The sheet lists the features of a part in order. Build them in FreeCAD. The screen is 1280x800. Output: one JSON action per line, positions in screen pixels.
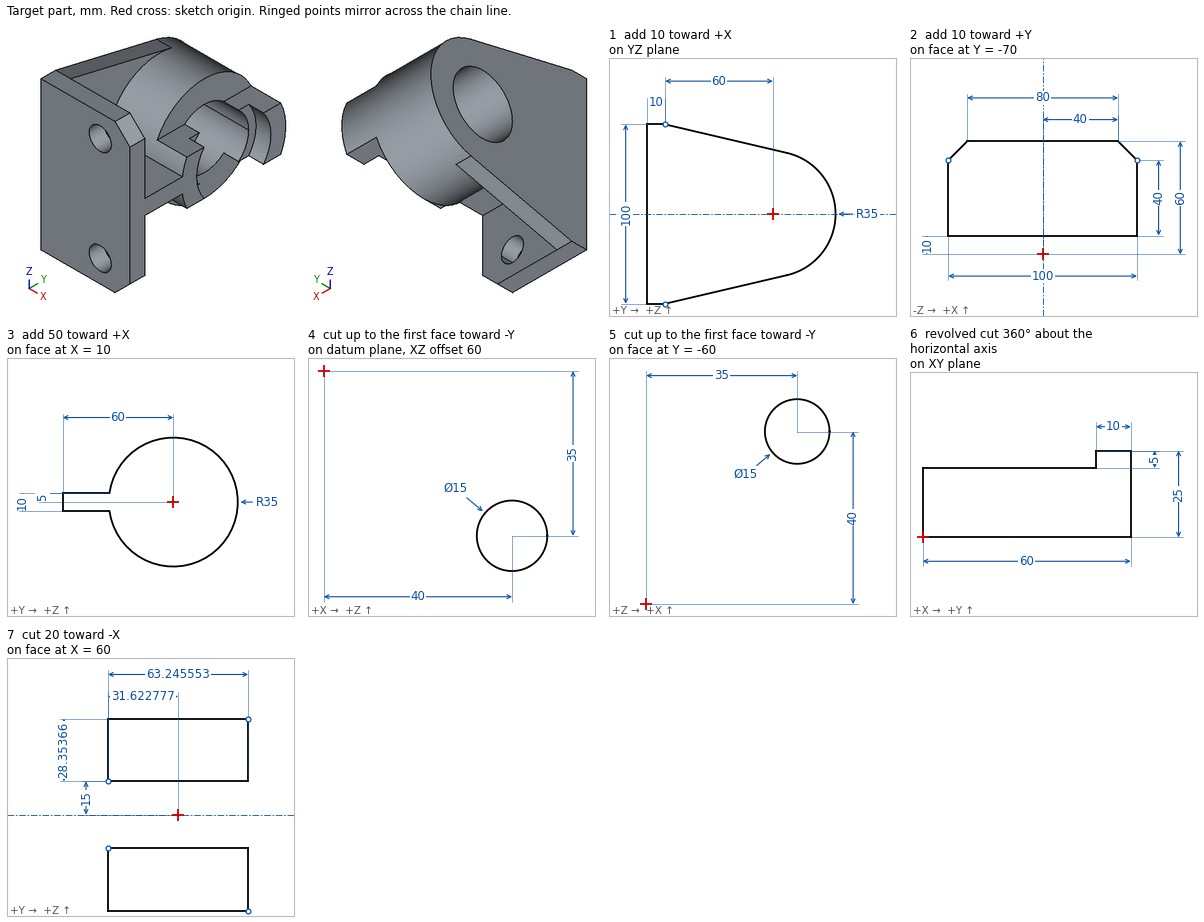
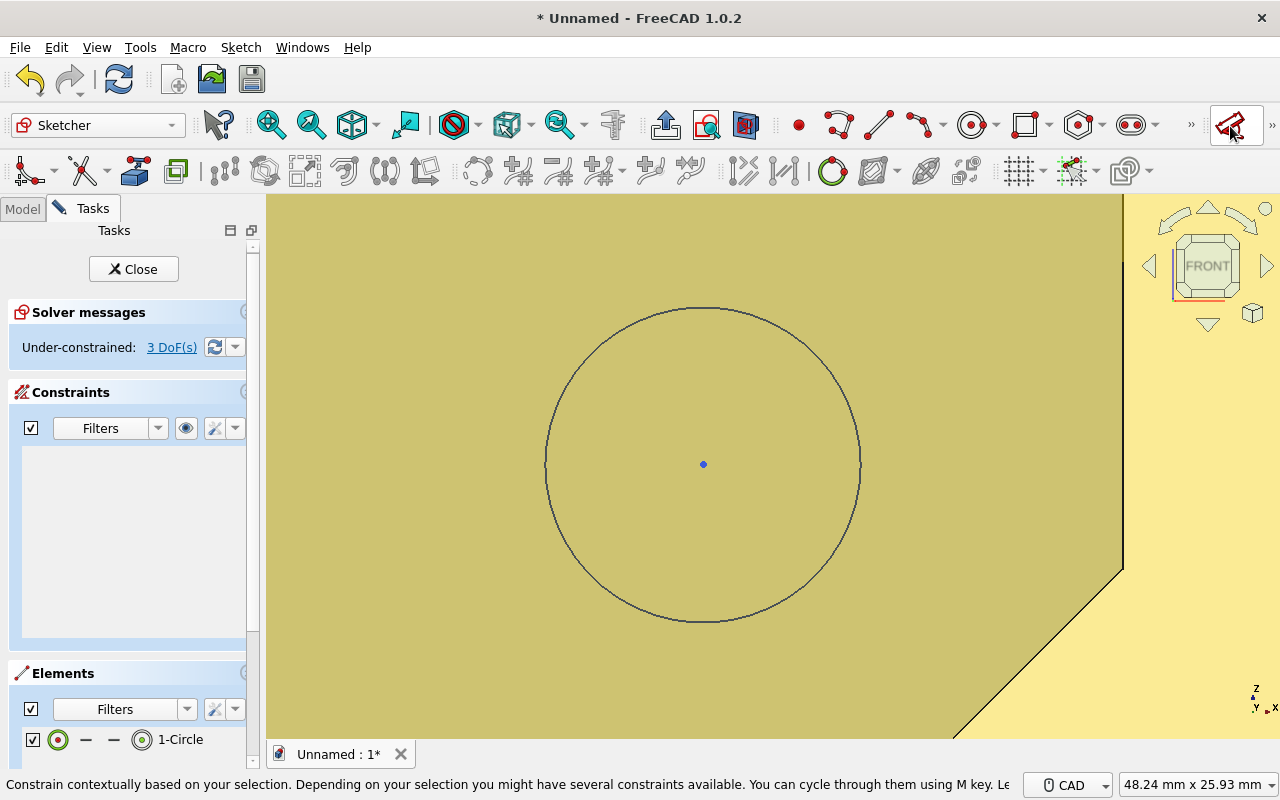
{"action": "left_click", "coordinate": [814, 353]}
{"action": "left_click", "coordinate": [837, 330]}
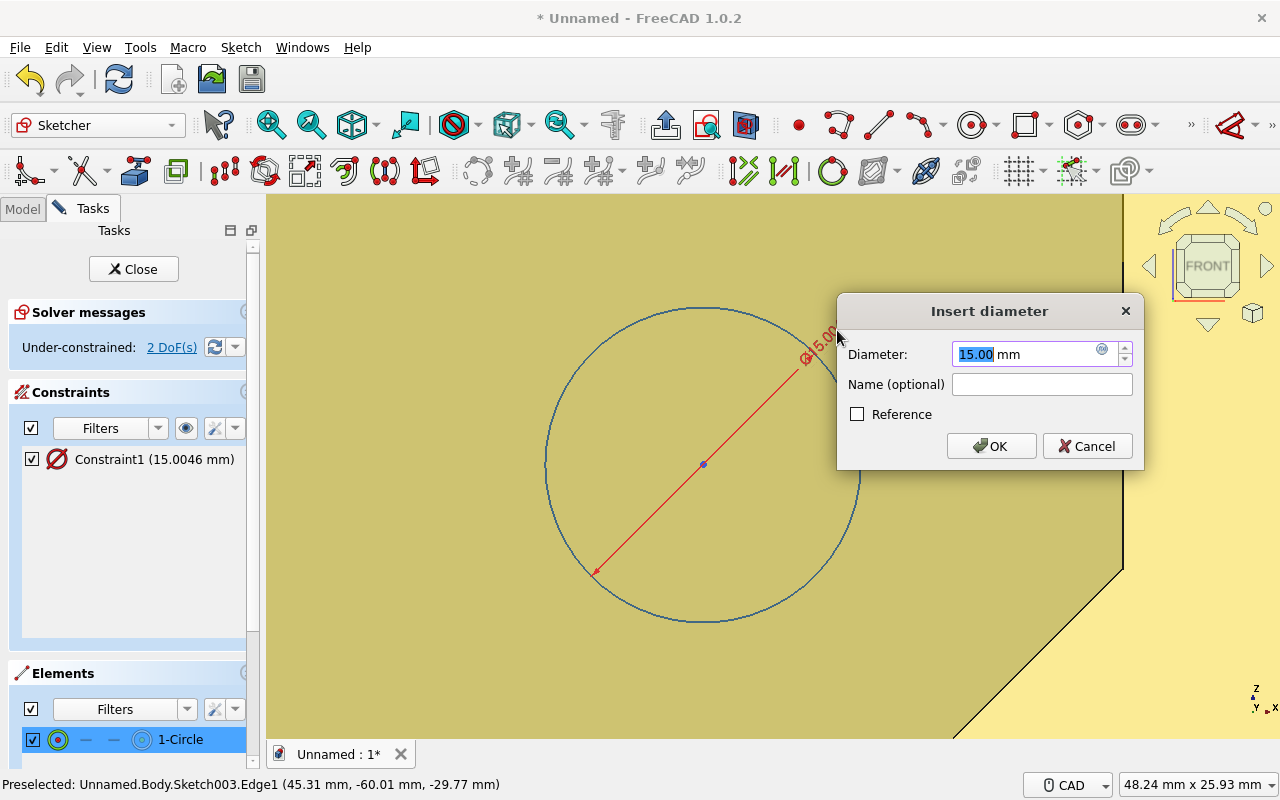
{"action": "type", "text": "15"}
{"action": "key", "text": "Return"}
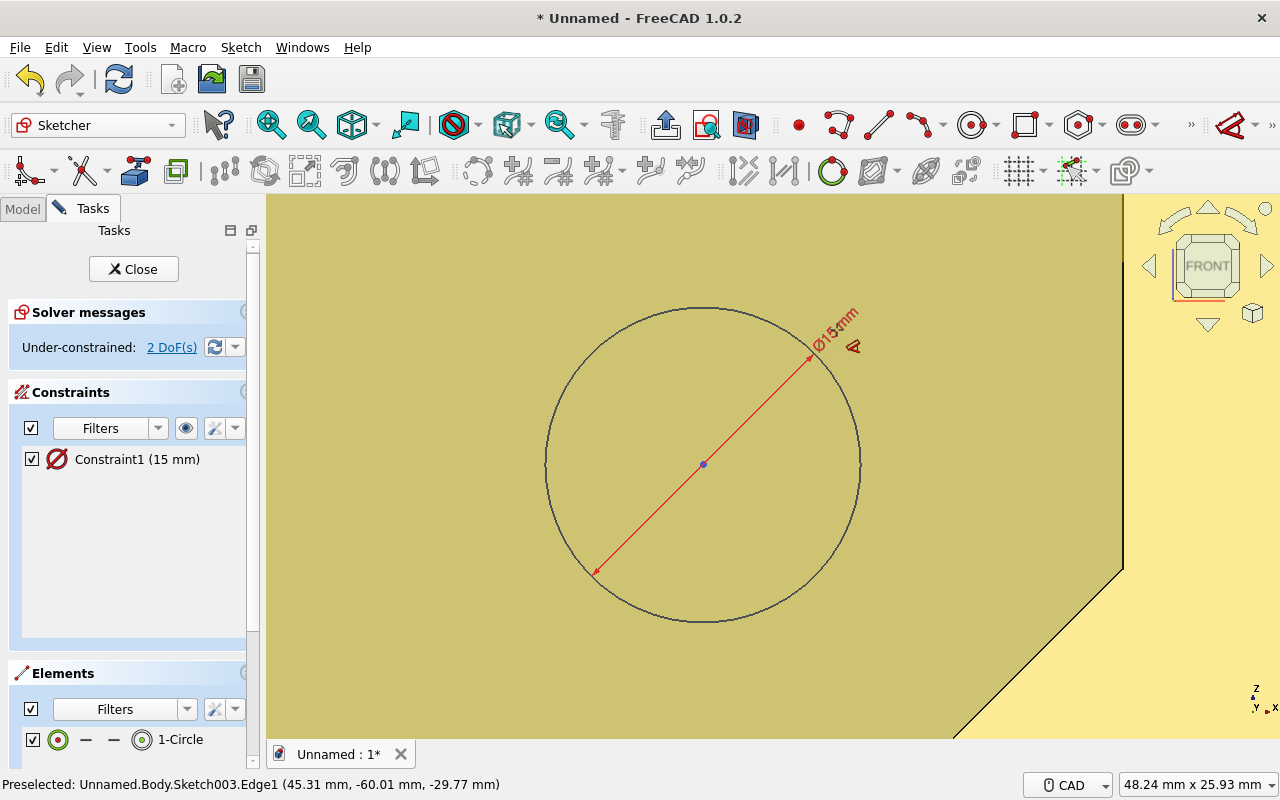
{"action": "left_click", "coordinate": [703, 465]}
{"action": "left_click", "coordinate": [498, 499]}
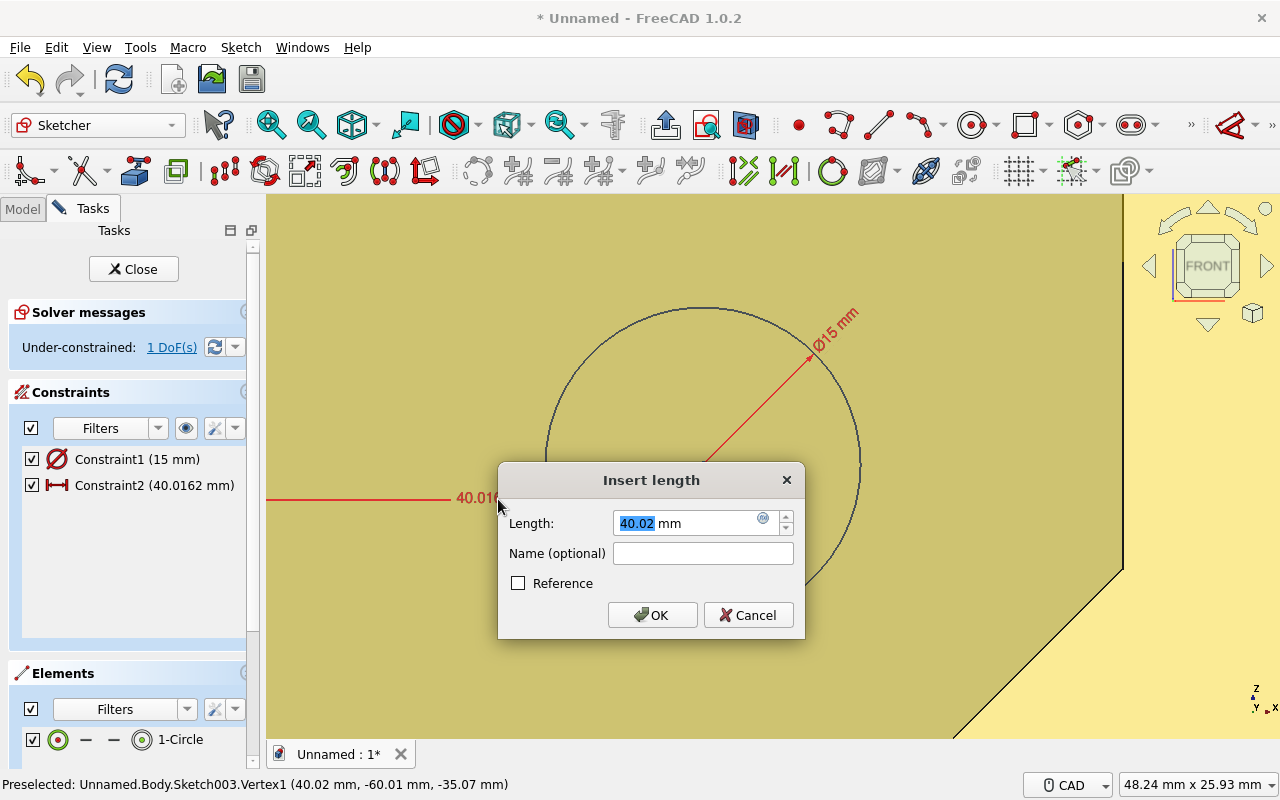
{"action": "type", "text": "40"}
{"action": "key", "text": "Return"}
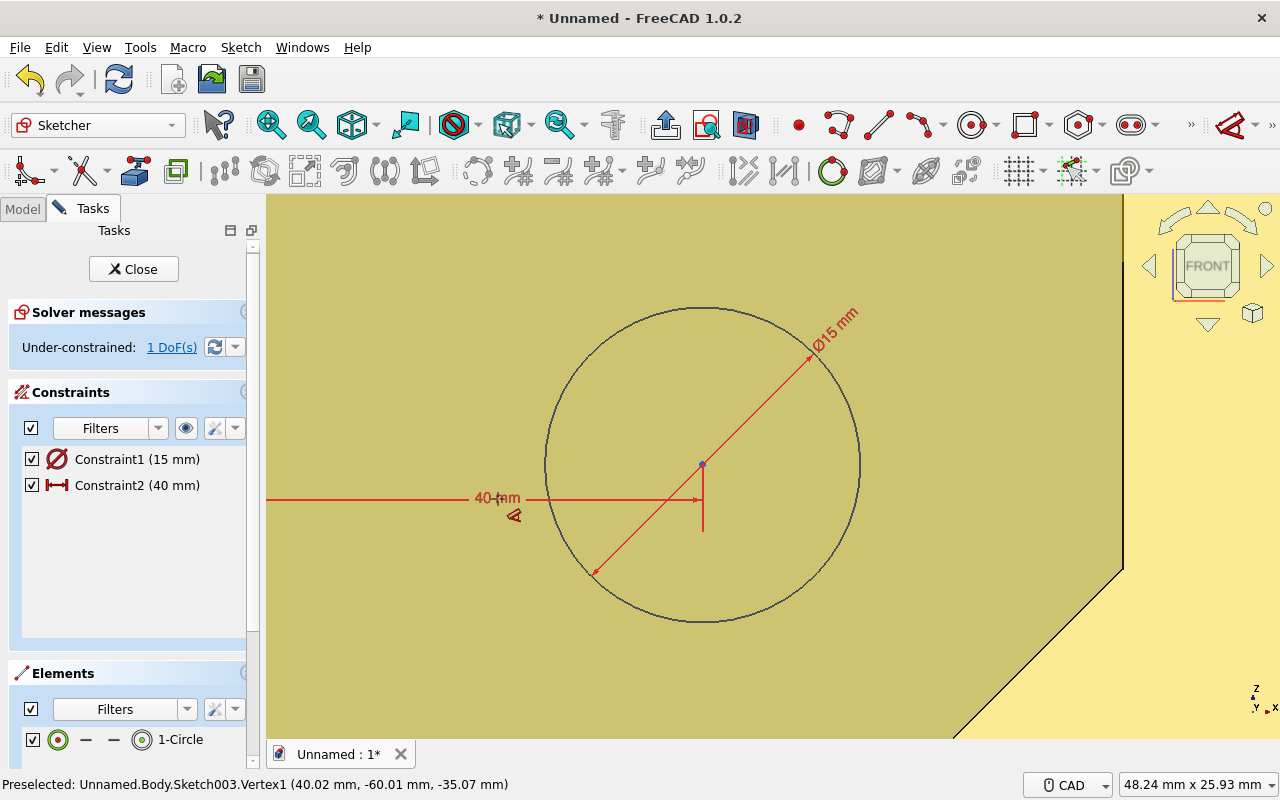
{"action": "left_click", "coordinate": [703, 465]}
{"action": "left_click", "coordinate": [737, 344]}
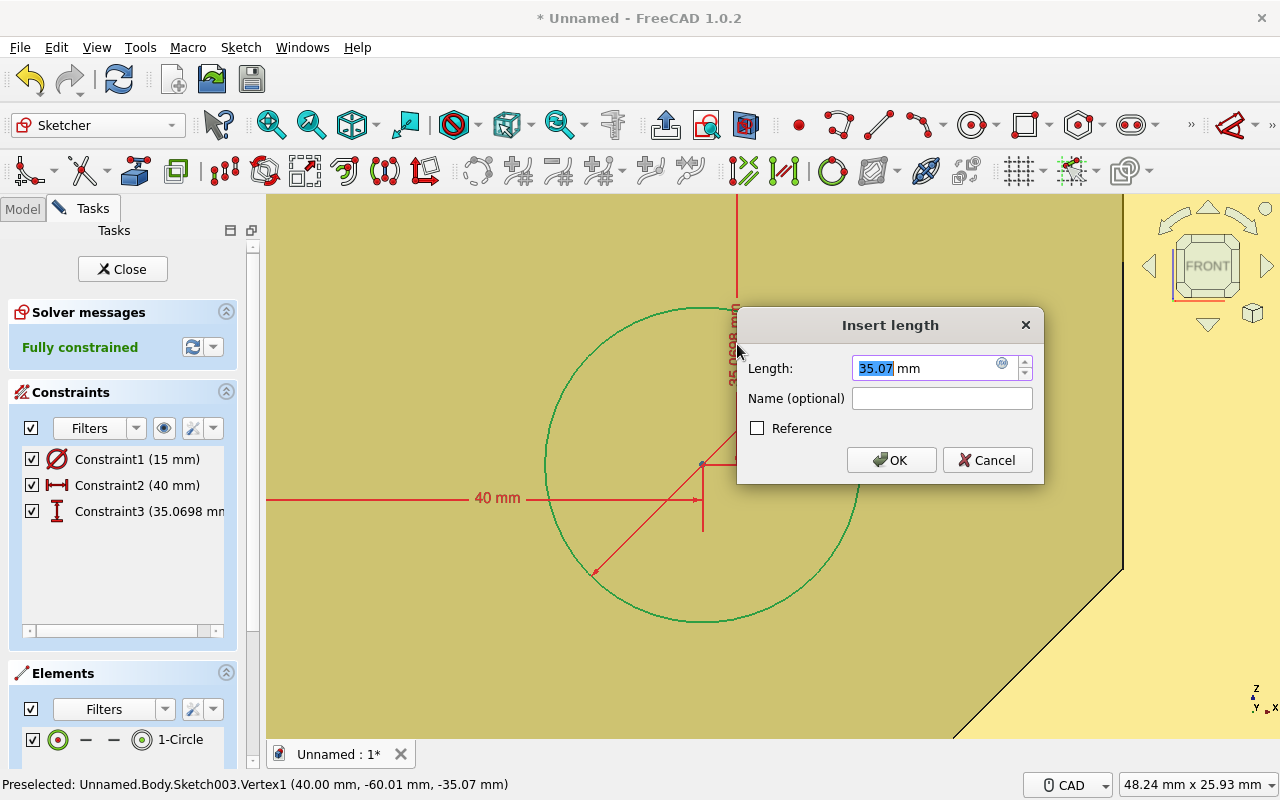
{"action": "type", "text": "35"}
{"action": "key", "text": "Return"}
{"action": "key", "text": "Escape"}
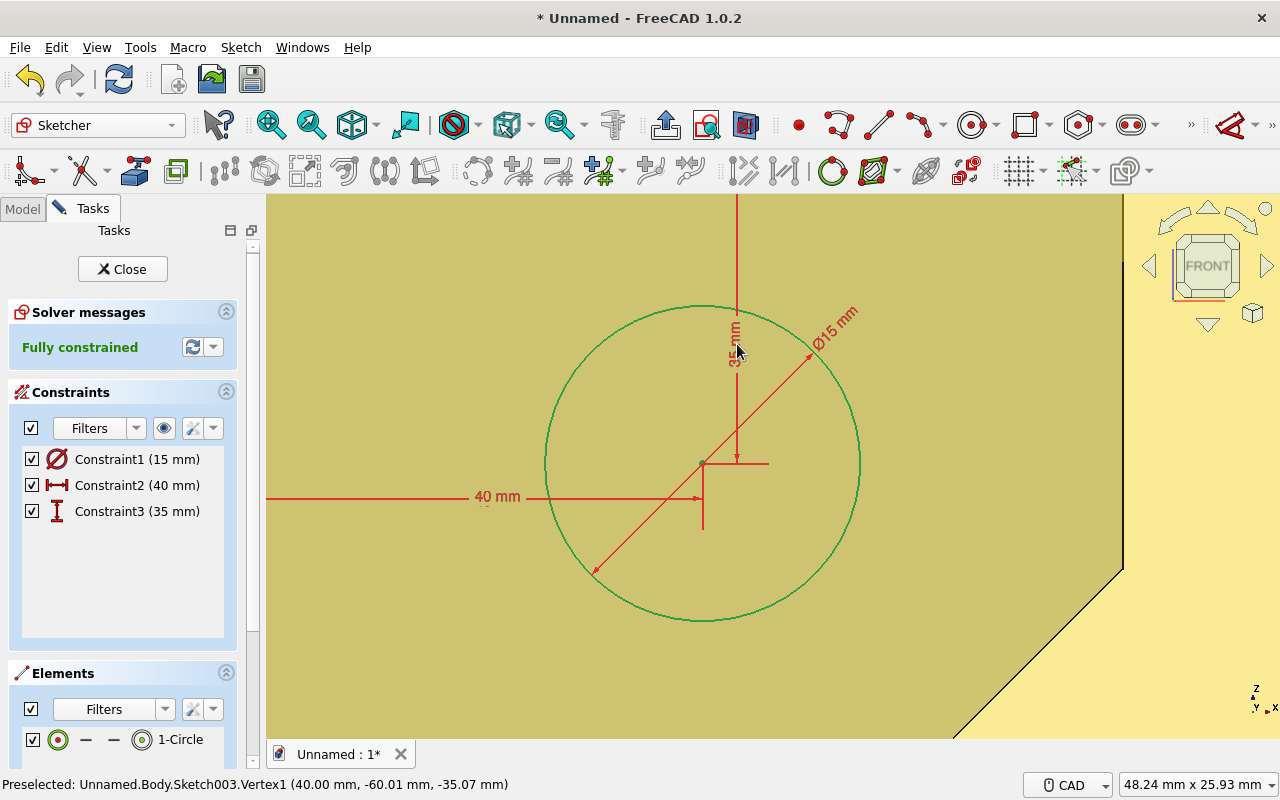
{"action": "left_click", "coordinate": [123, 269]}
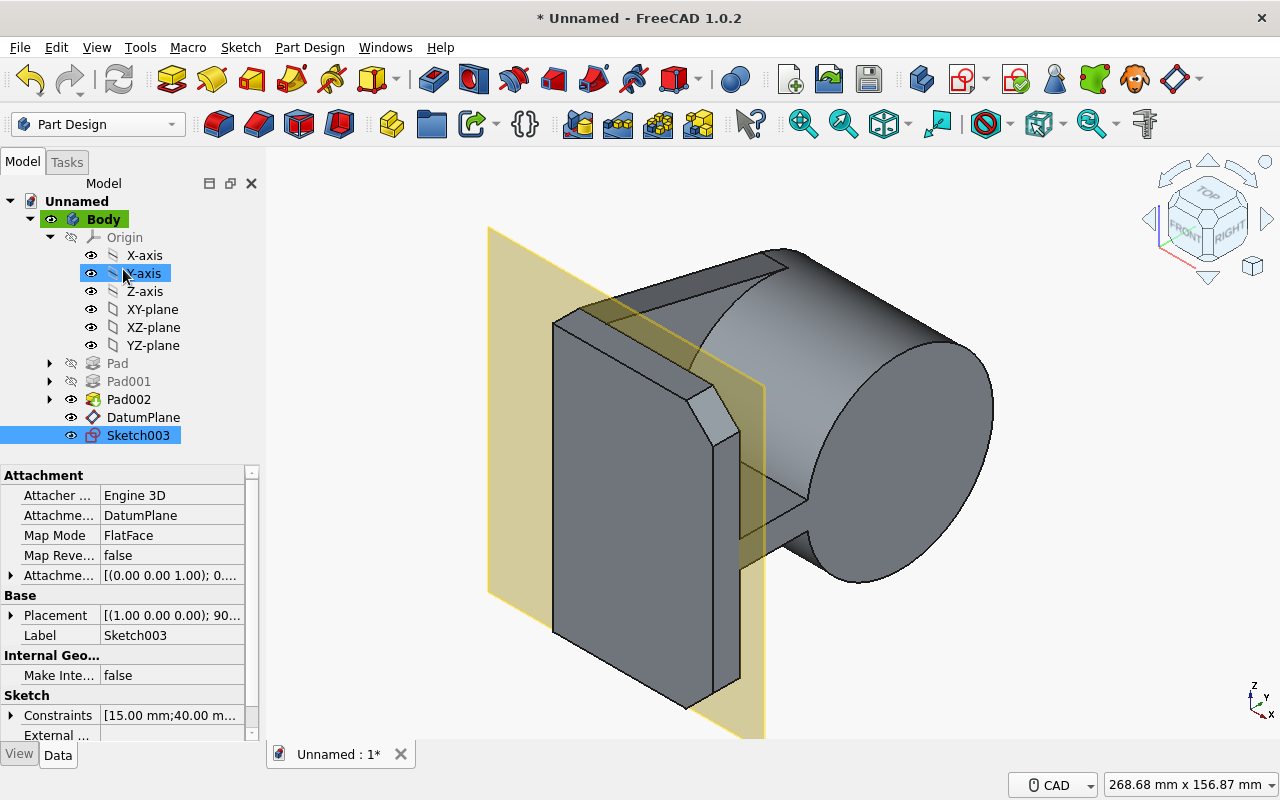
{"action": "left_click", "coordinate": [434, 80]}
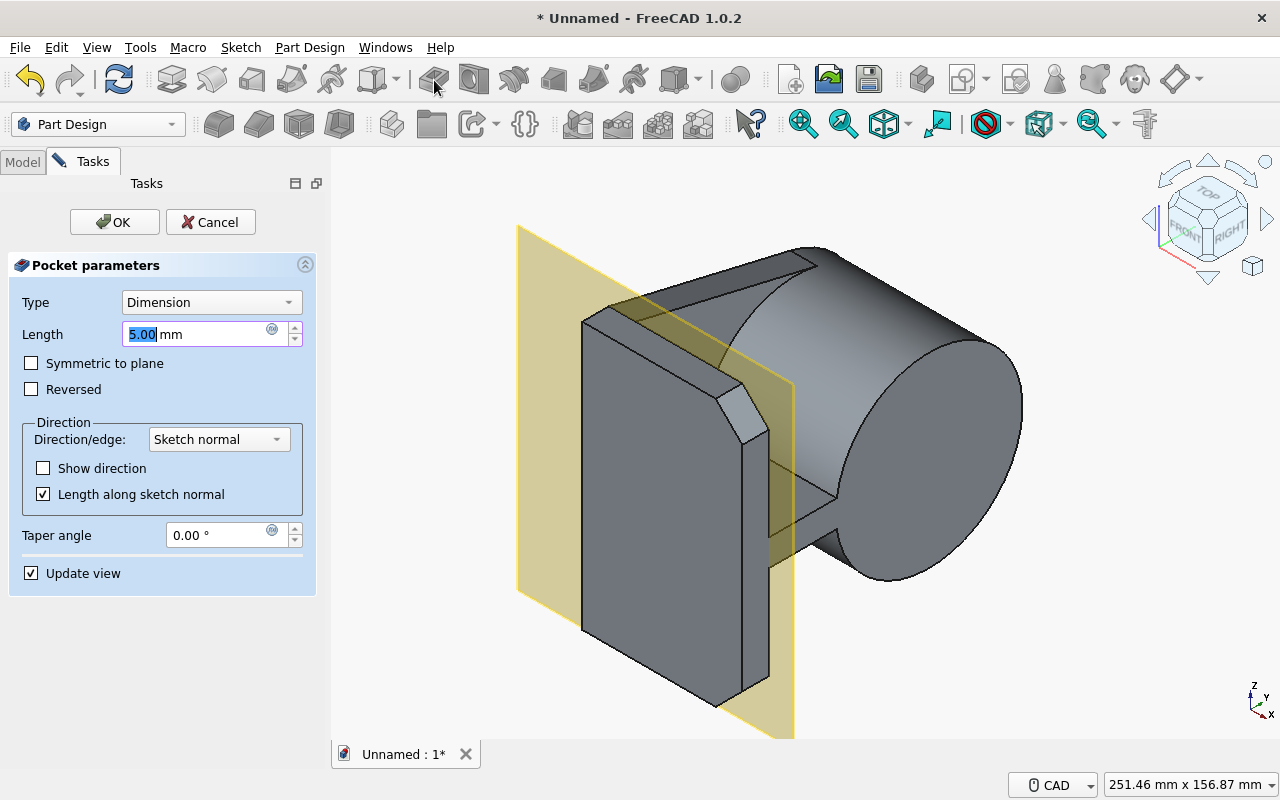
{"action": "left_click", "coordinate": [212, 302]}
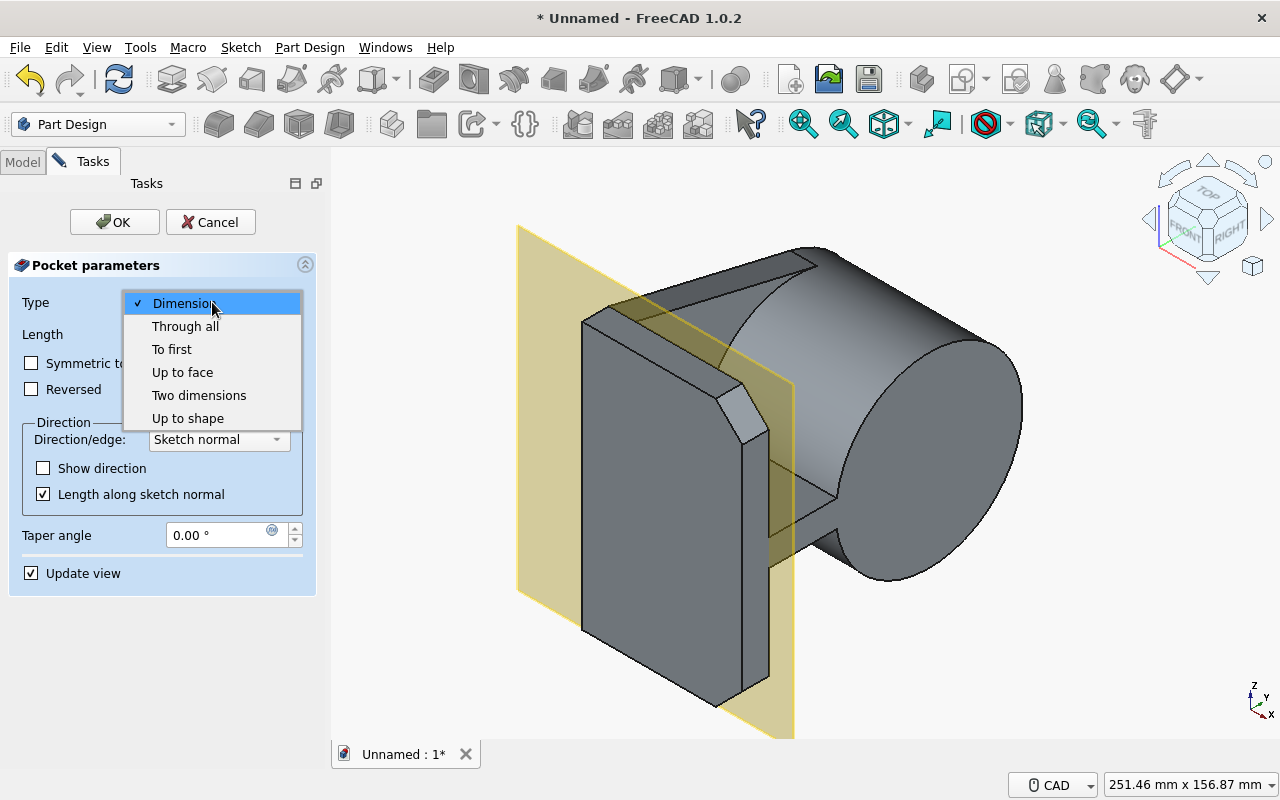
{"action": "left_click", "coordinate": [212, 350]}